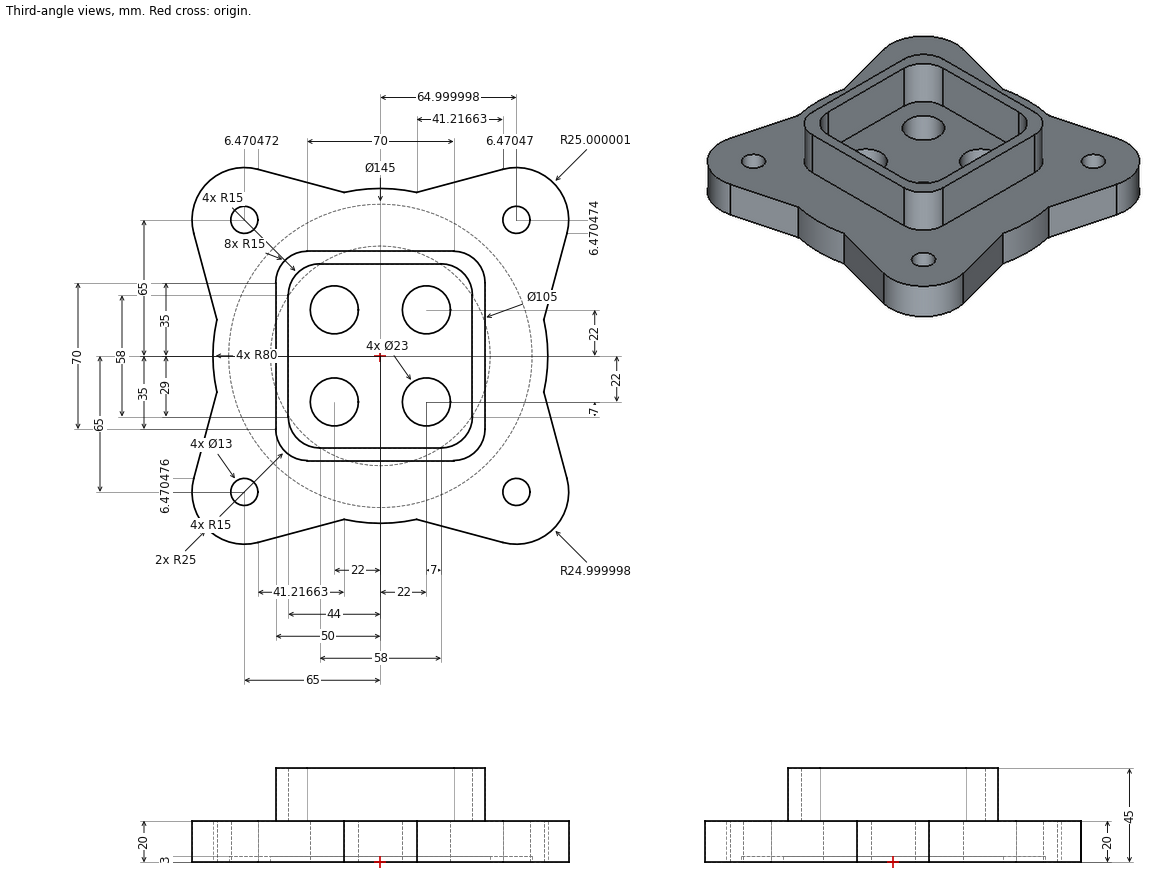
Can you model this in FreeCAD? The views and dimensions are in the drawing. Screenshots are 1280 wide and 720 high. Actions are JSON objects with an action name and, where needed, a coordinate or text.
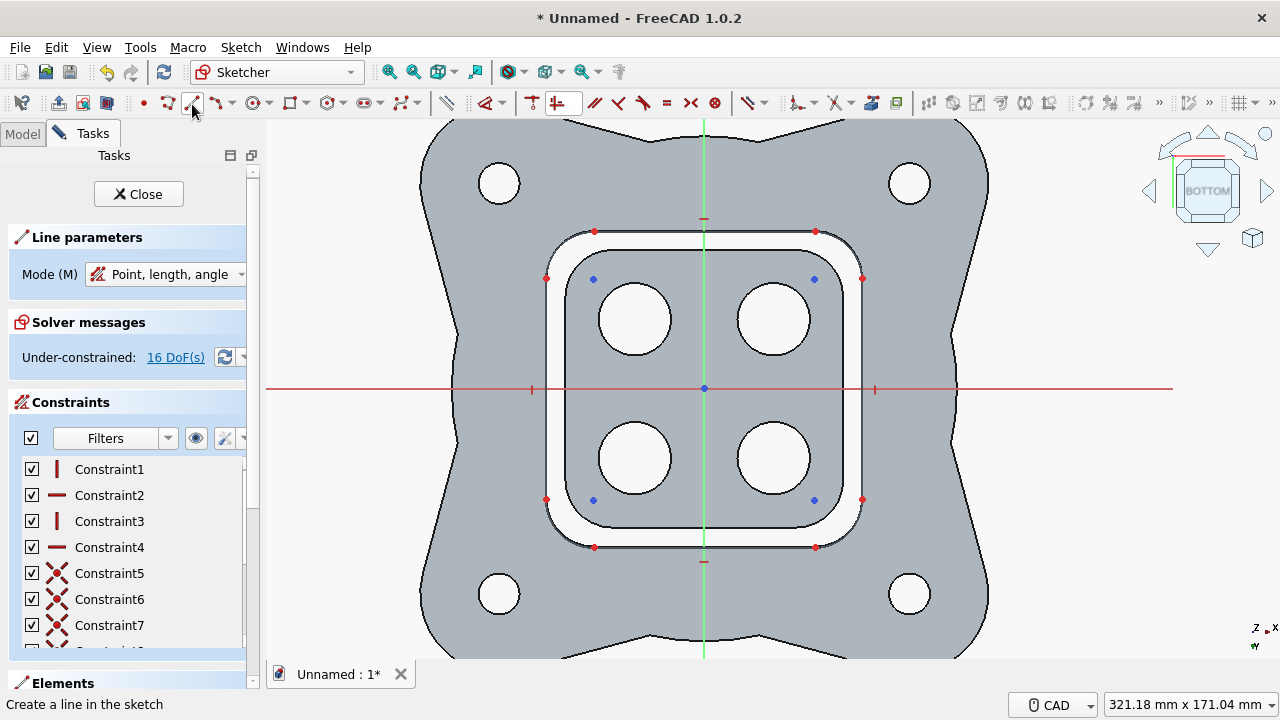
{"action": "left_click", "coordinate": [565, 297]}
{"action": "left_click", "coordinate": [565, 480]}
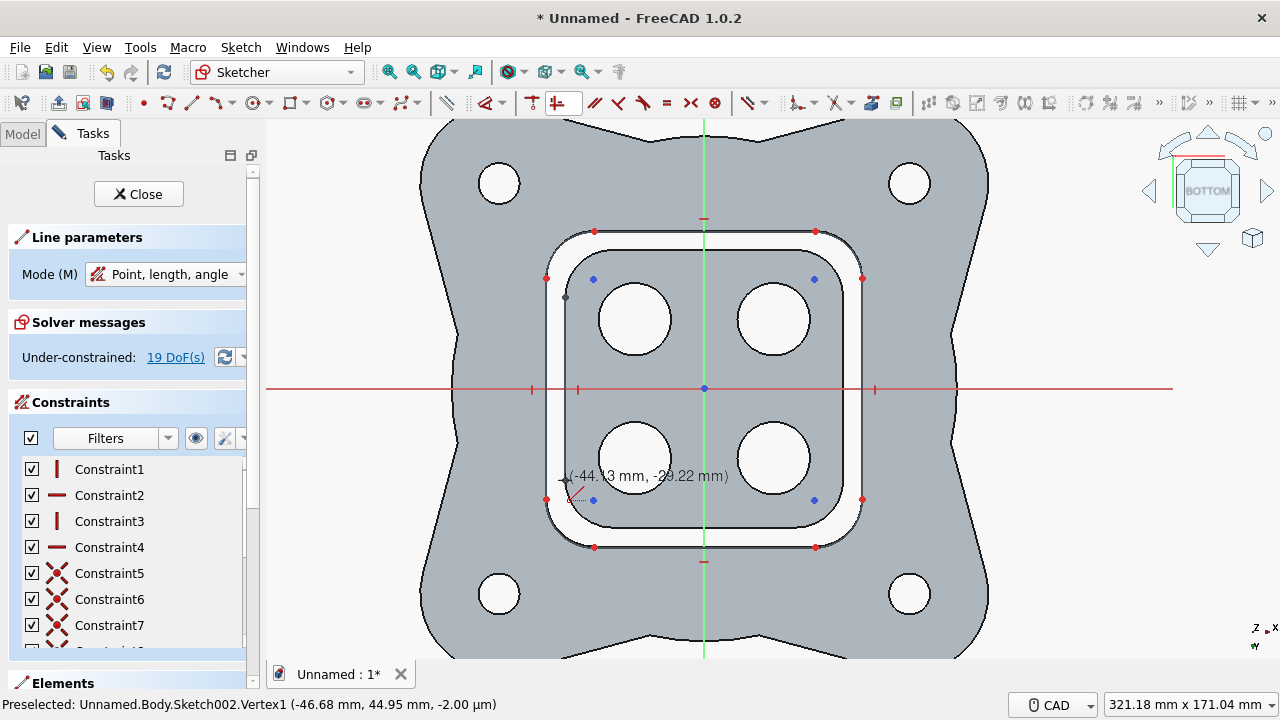
{"action": "left_click", "coordinate": [613, 528]}
{"action": "left_click", "coordinate": [796, 528]}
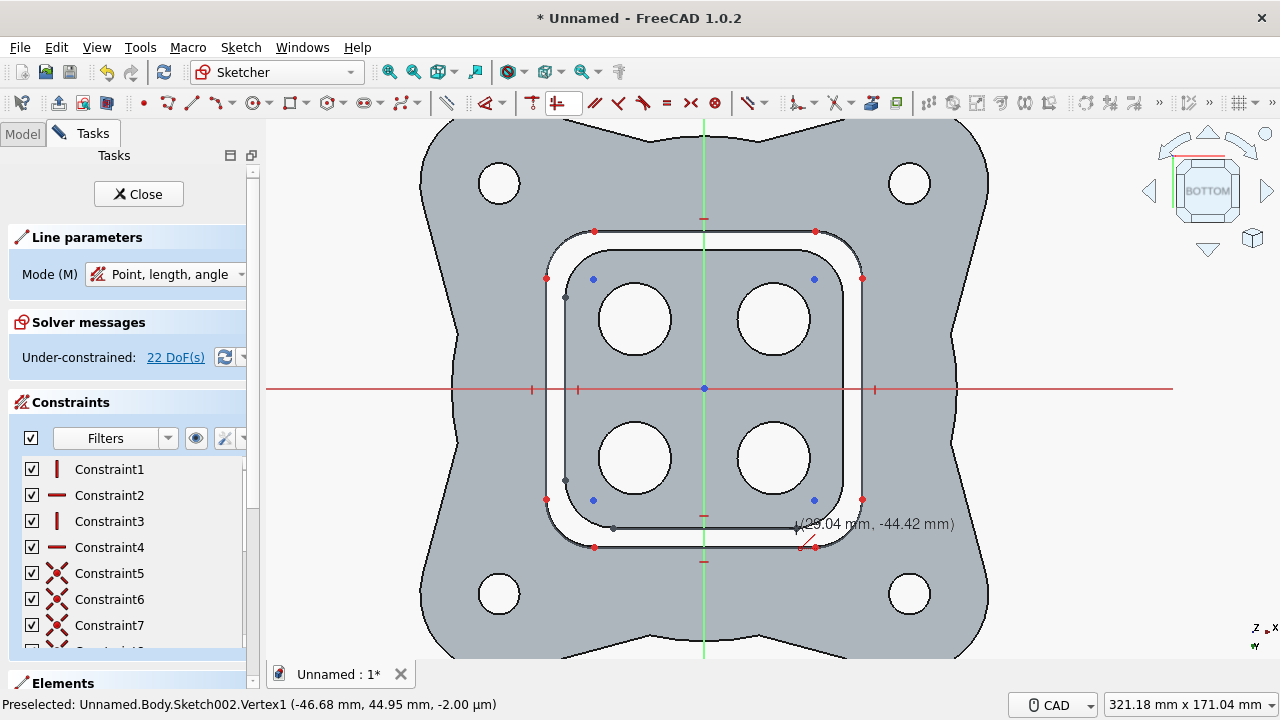
{"action": "left_click", "coordinate": [843, 480]}
{"action": "left_click", "coordinate": [843, 297]}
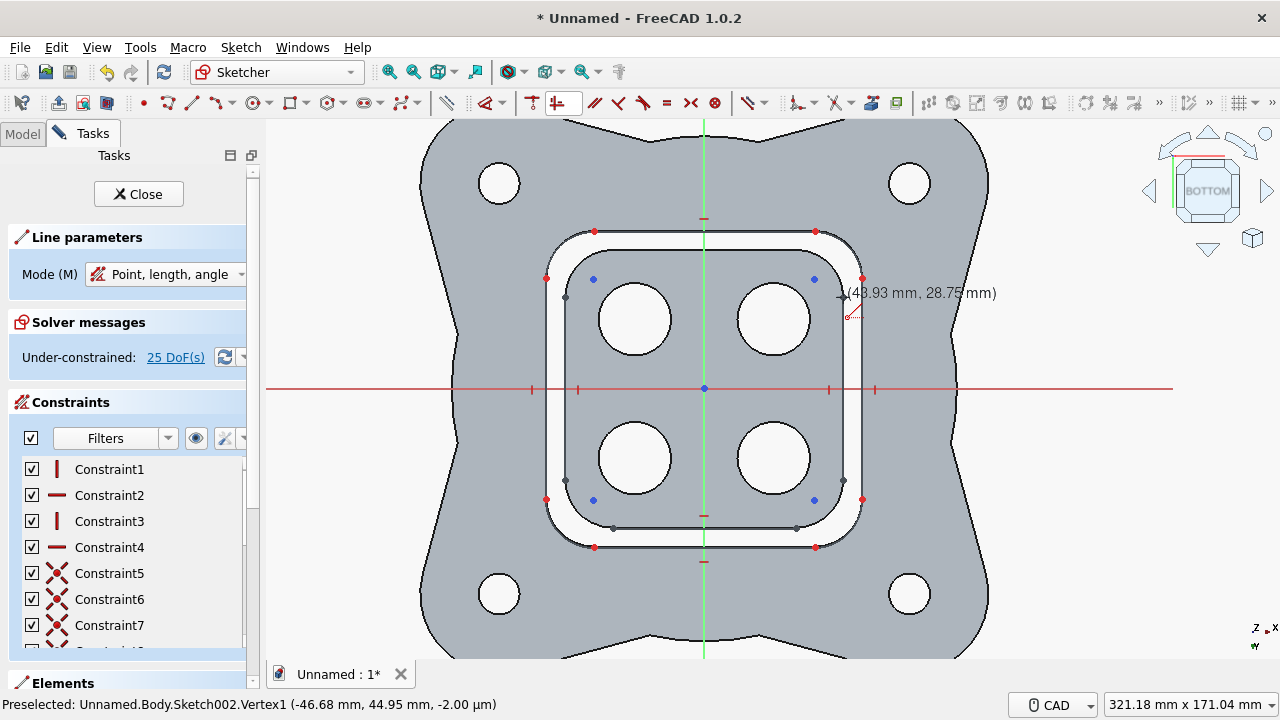
{"action": "left_click", "coordinate": [796, 250]}
{"action": "left_click", "coordinate": [613, 250]}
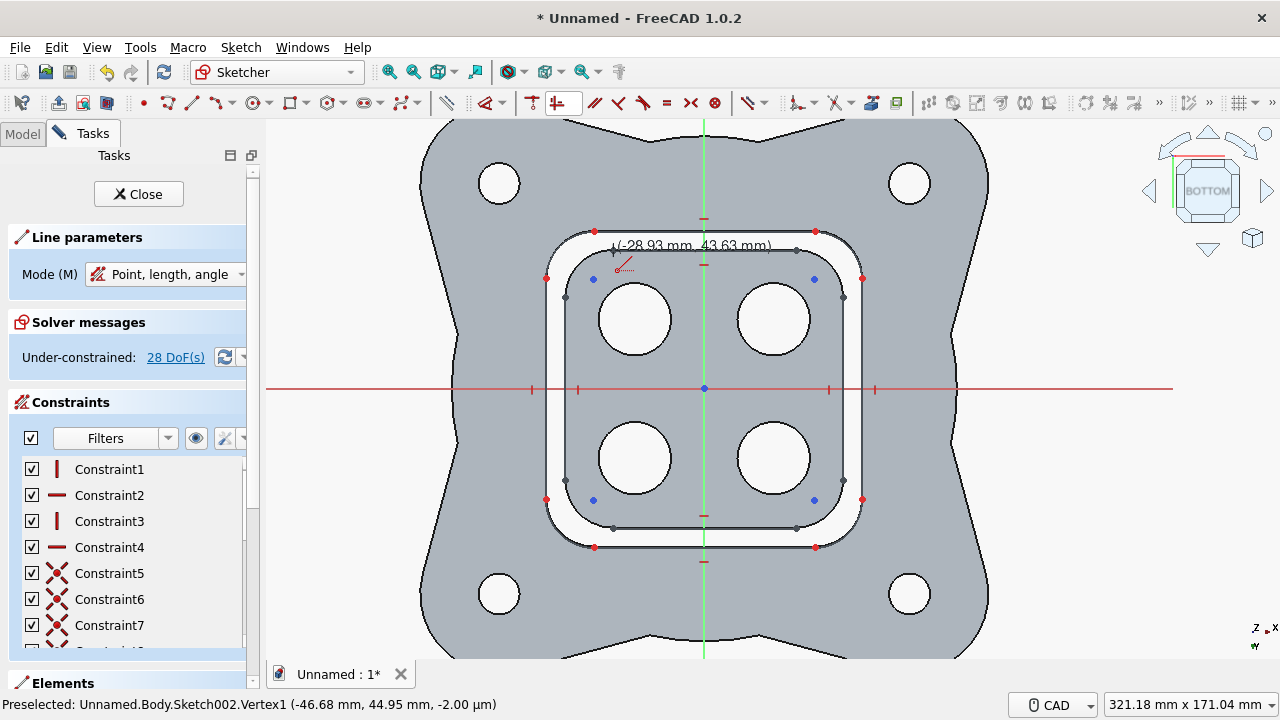
{"action": "key", "text": "g 3 a"}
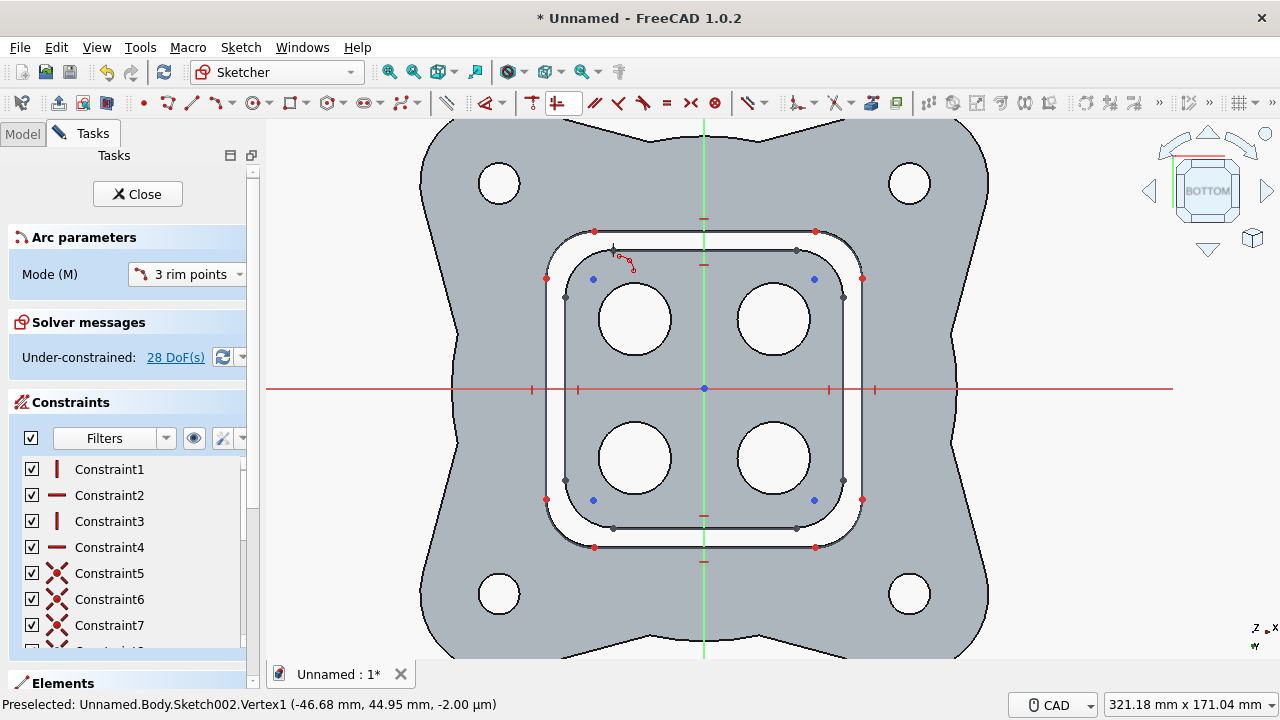
{"action": "left_click", "coordinate": [565, 481]}
{"action": "left_click", "coordinate": [613, 529]}
{"action": "left_click", "coordinate": [579, 514]}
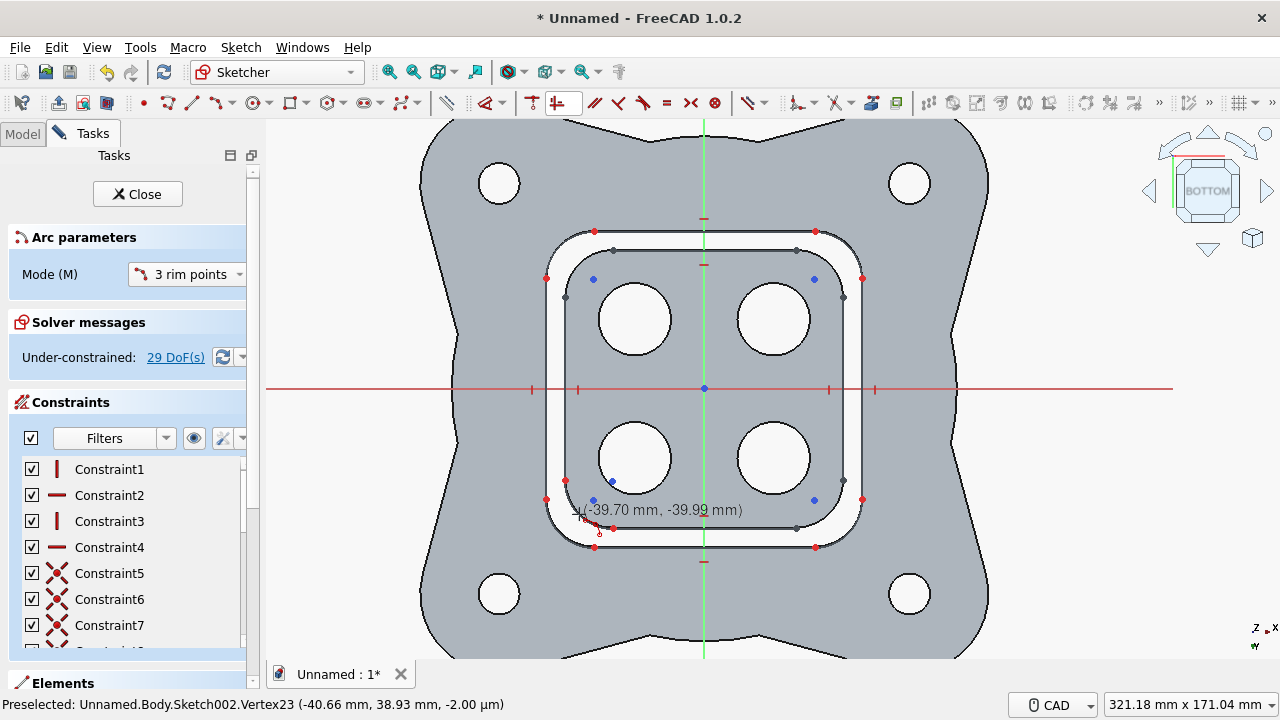
{"action": "left_click", "coordinate": [796, 529]}
{"action": "left_click", "coordinate": [843, 481]}
{"action": "left_click", "coordinate": [829, 514]}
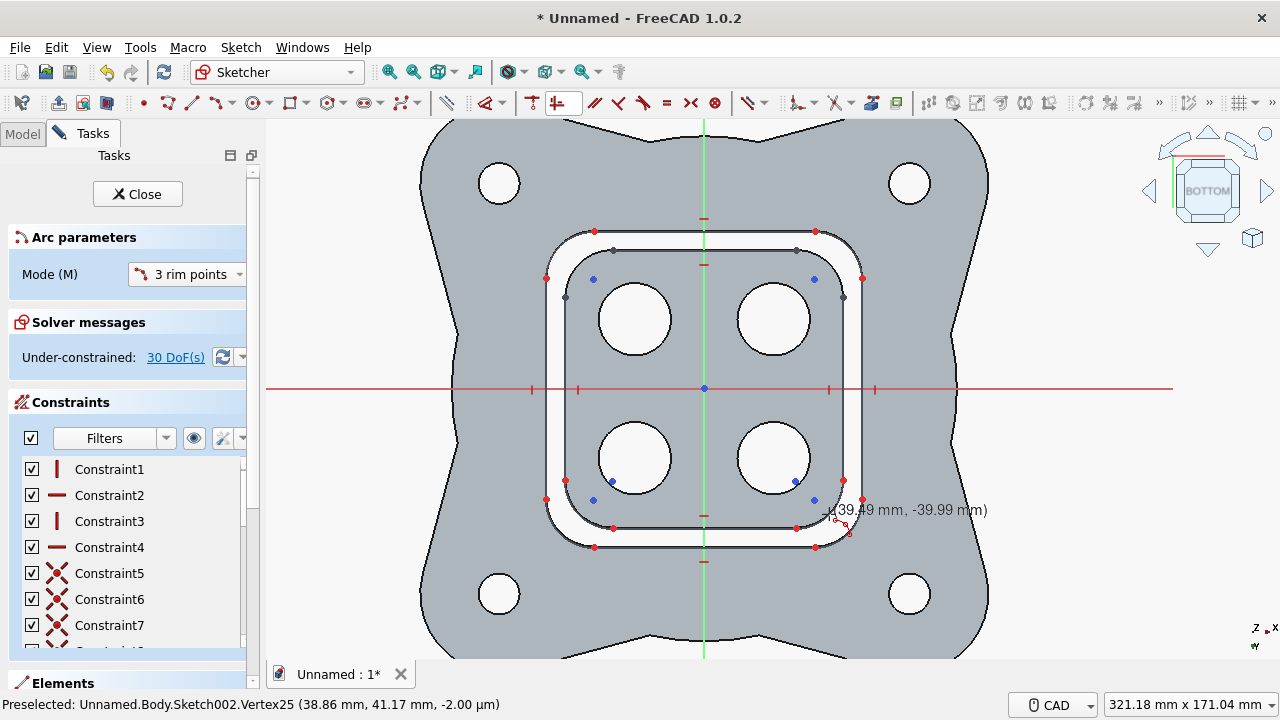
{"action": "left_click", "coordinate": [843, 298]}
{"action": "left_click", "coordinate": [796, 251]}
{"action": "left_click", "coordinate": [829, 264]}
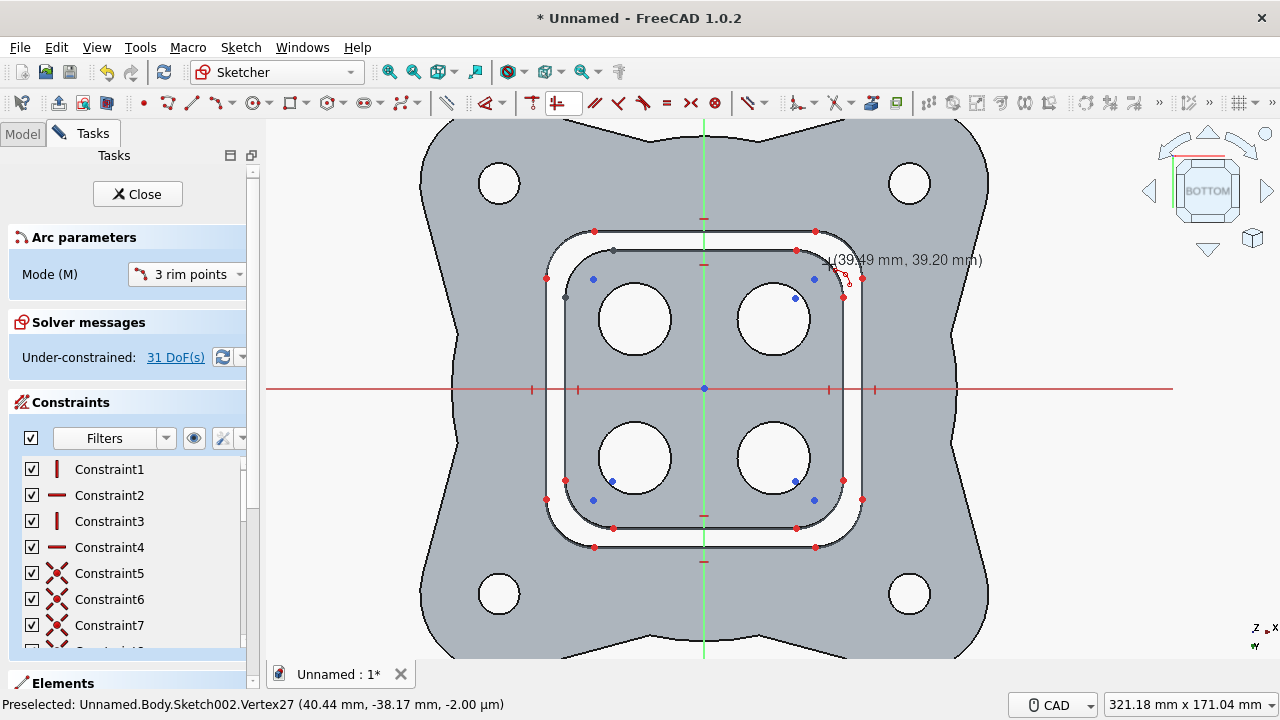
{"action": "left_click", "coordinate": [613, 251]}
{"action": "left_click", "coordinate": [565, 298]}
{"action": "left_click", "coordinate": [579, 264]}
{"action": "key", "text": "Escape"}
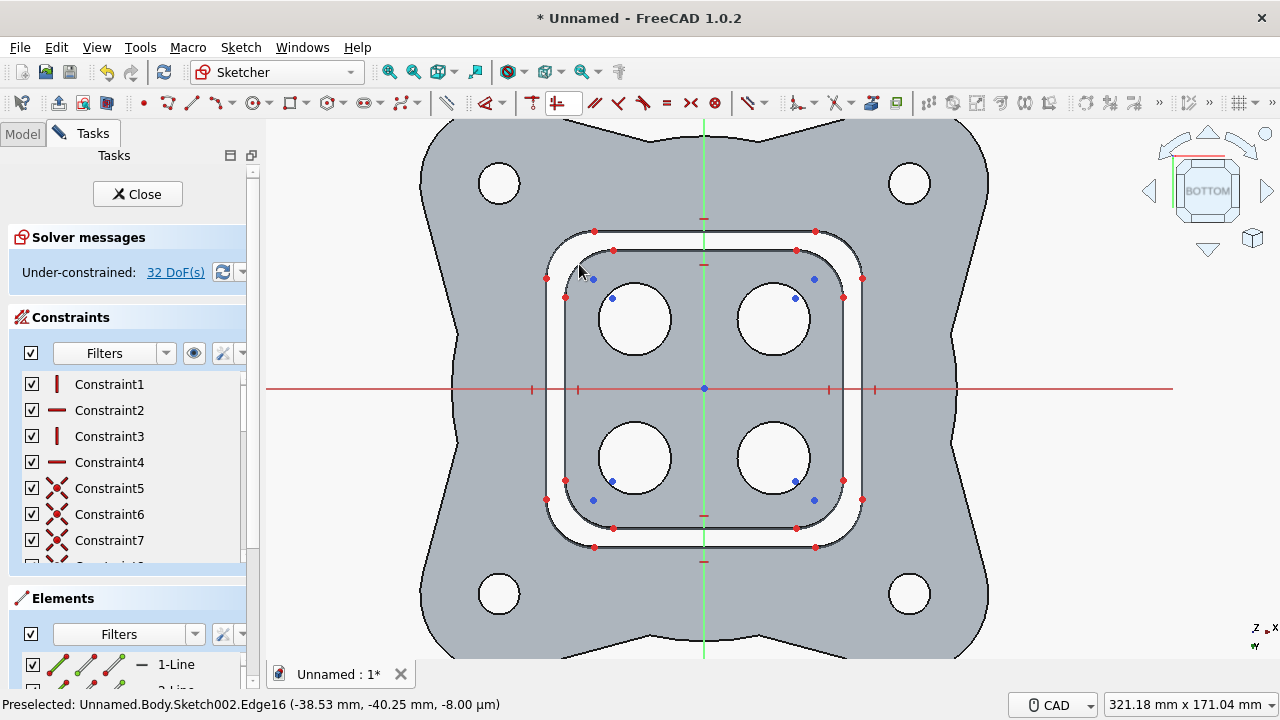
{"action": "left_click", "coordinate": [546, 434]}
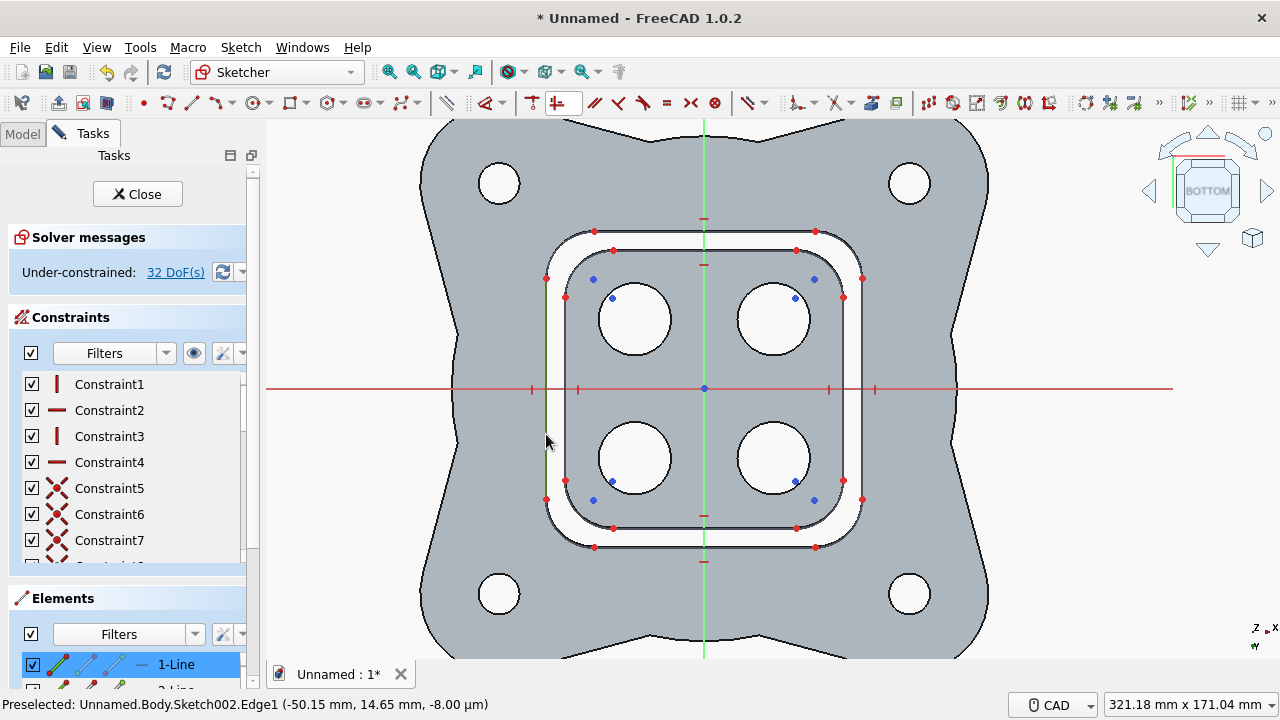
{"action": "left_click", "coordinate": [572, 237]}